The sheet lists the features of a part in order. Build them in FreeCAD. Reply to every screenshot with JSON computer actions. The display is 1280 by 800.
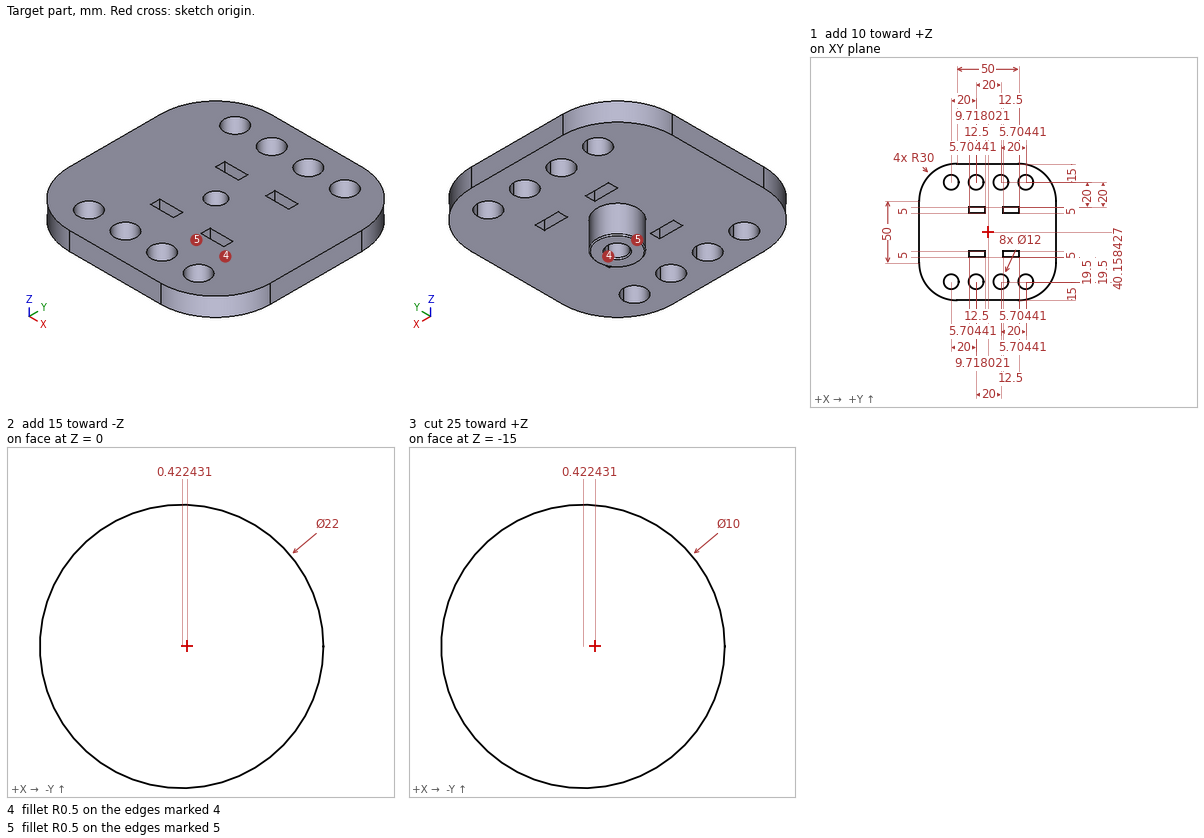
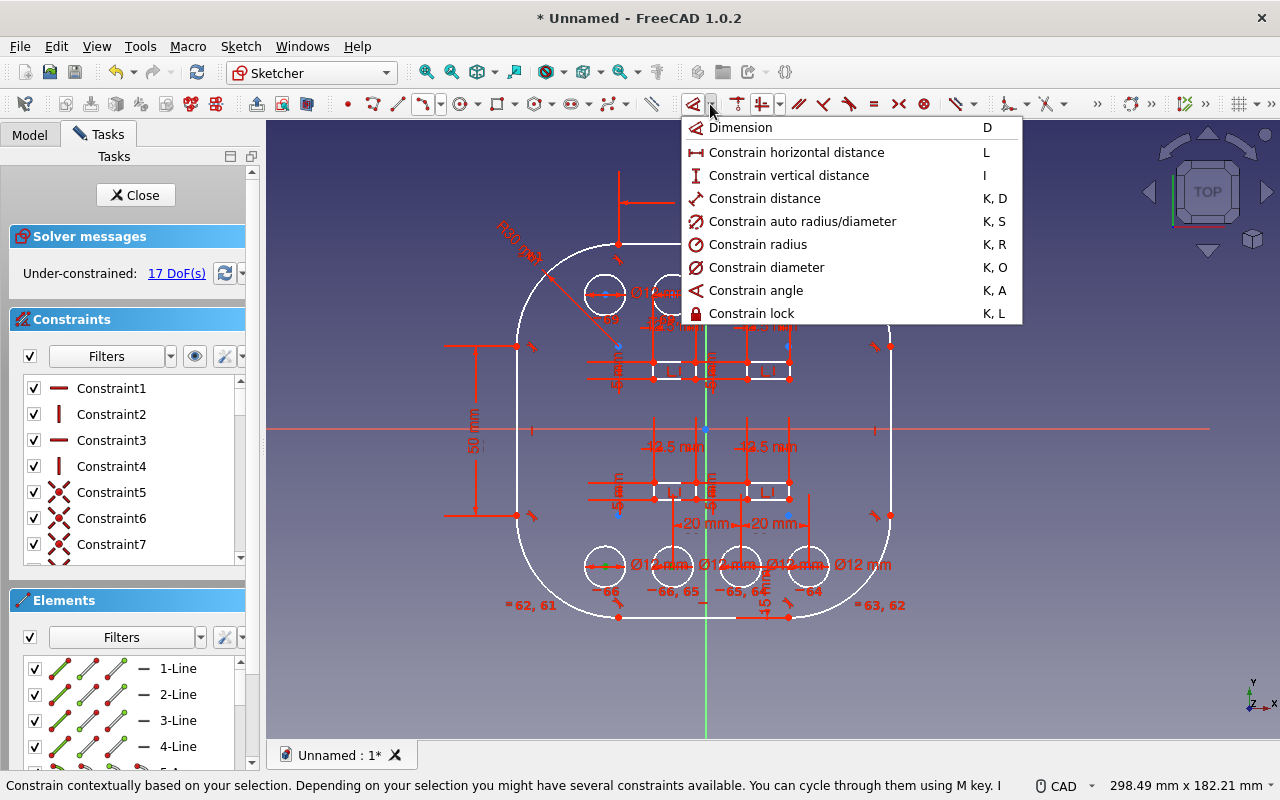
{"action": "left_click", "coordinate": [852, 152]}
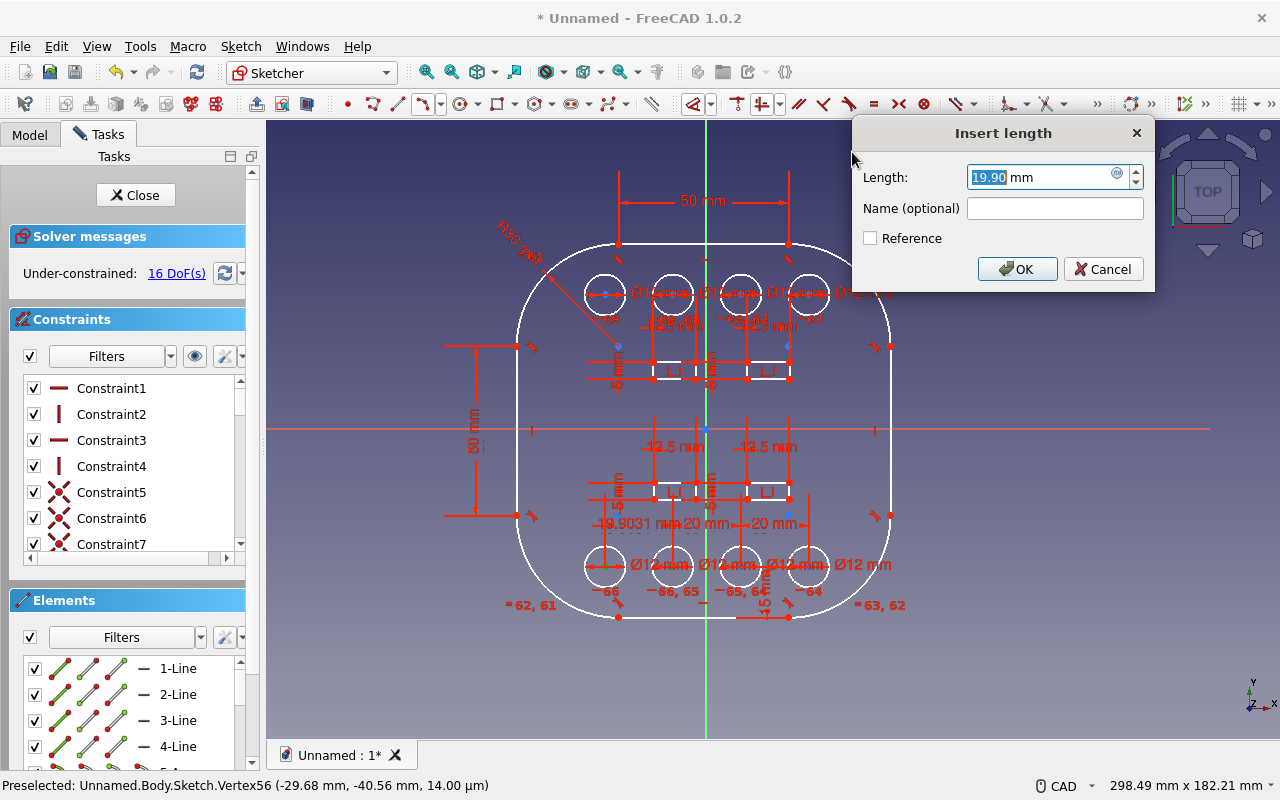
{"action": "type", "text": "20"}
{"action": "key", "text": "Return"}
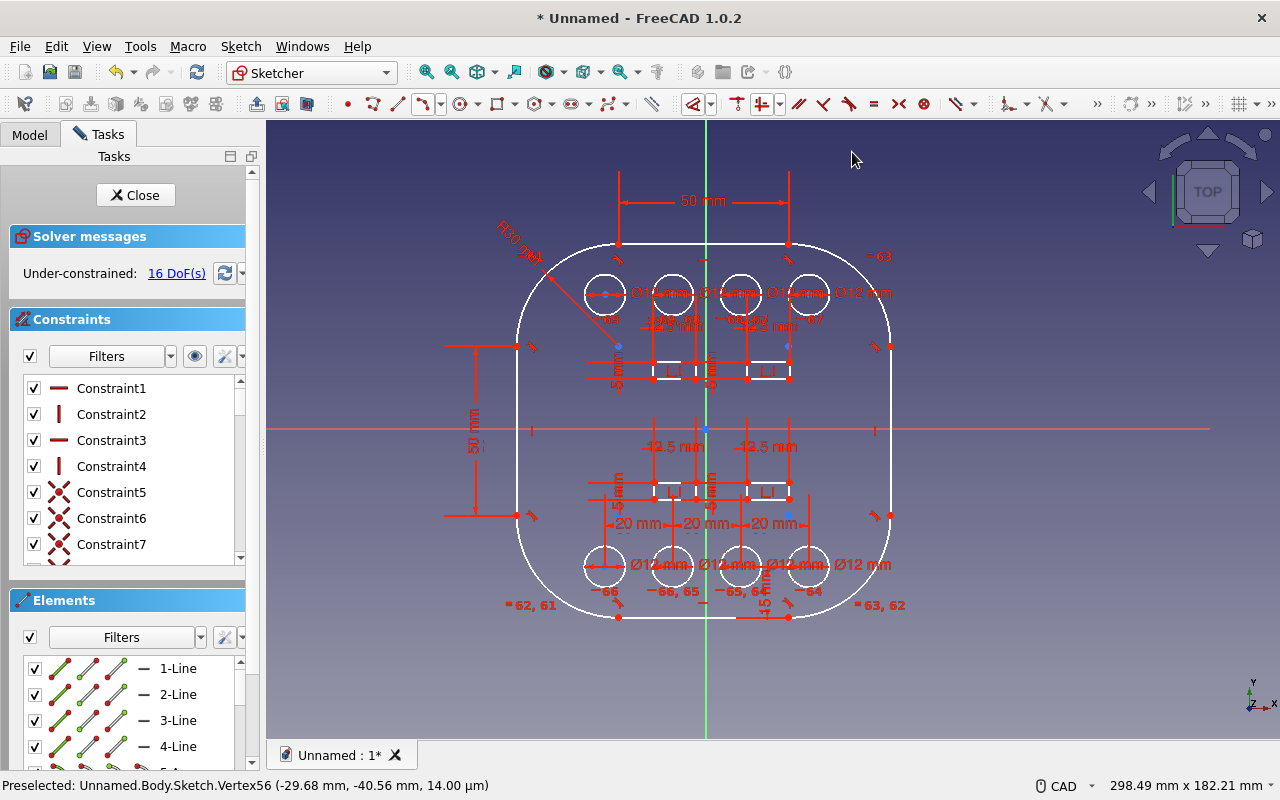
{"action": "left_click", "coordinate": [789, 244]}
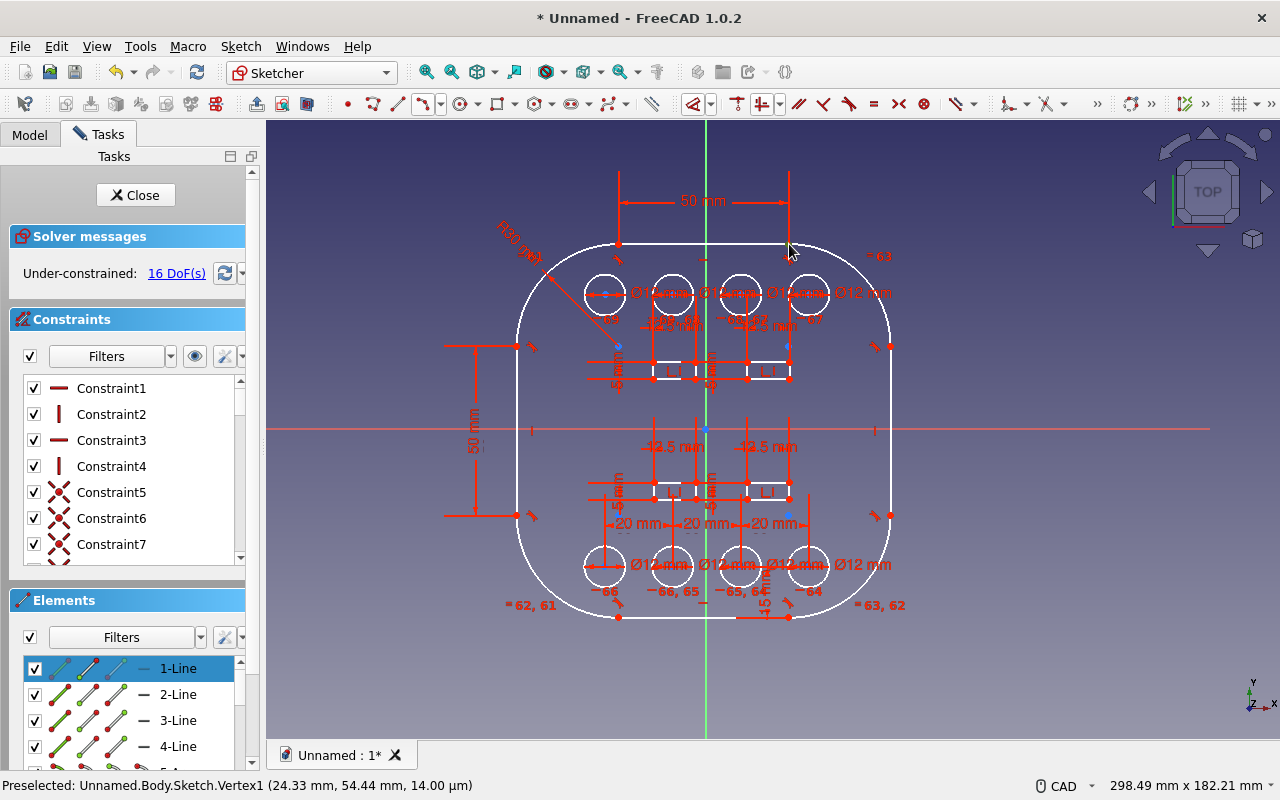
{"action": "left_click", "coordinate": [809, 295]}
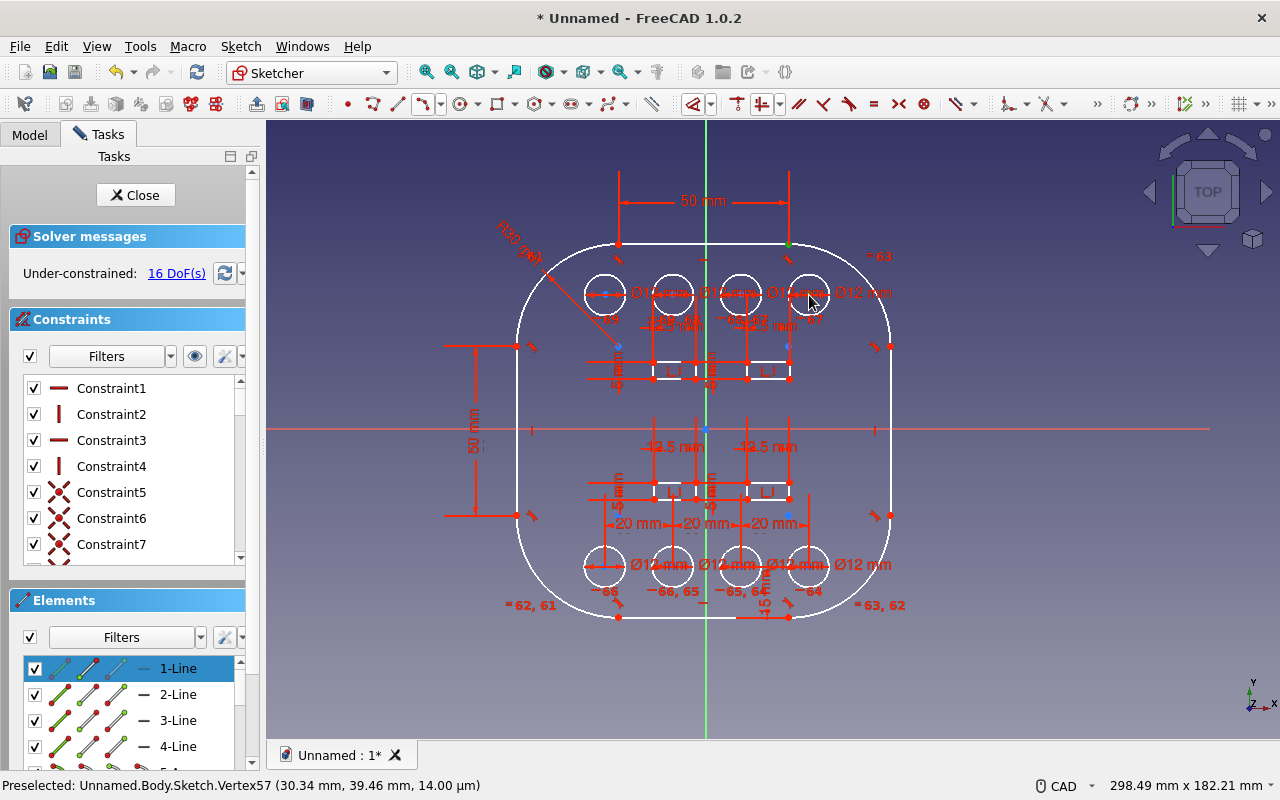
{"action": "left_click", "coordinate": [710, 104]}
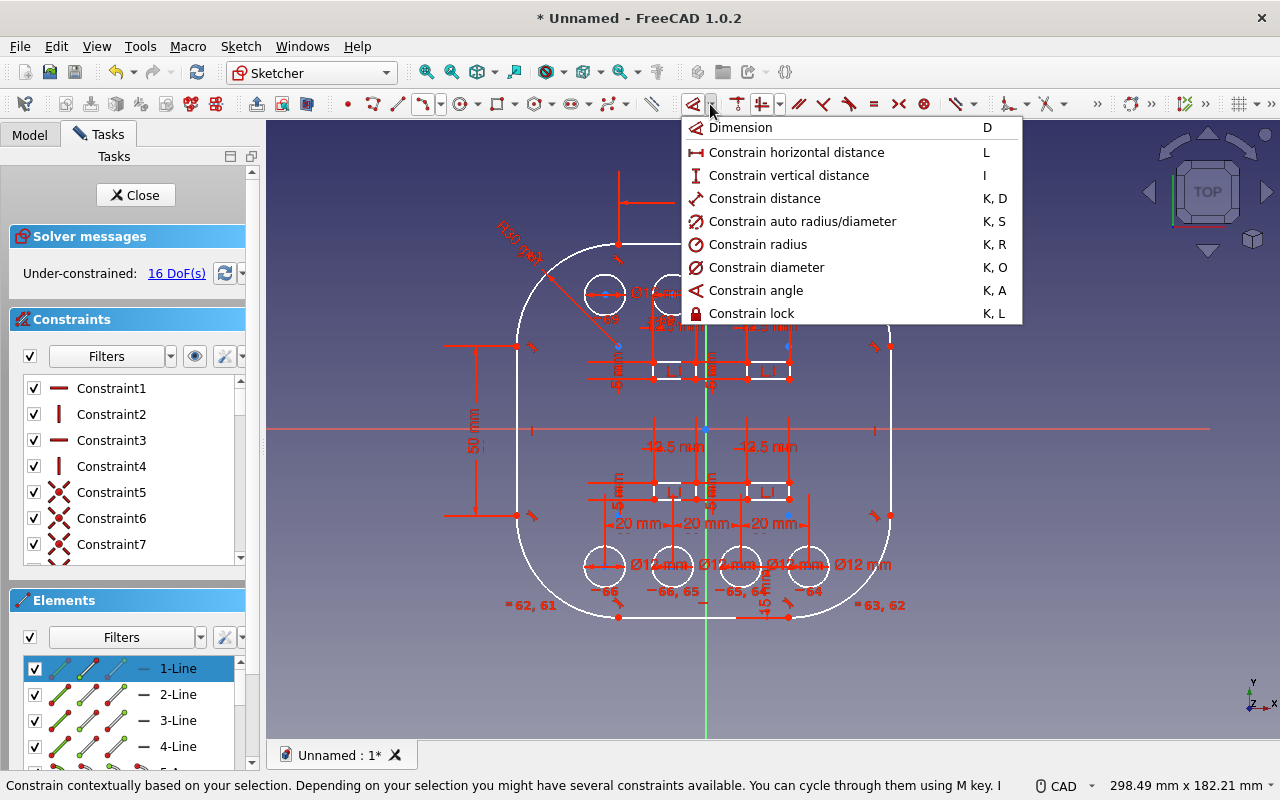
{"action": "left_click", "coordinate": [852, 176]}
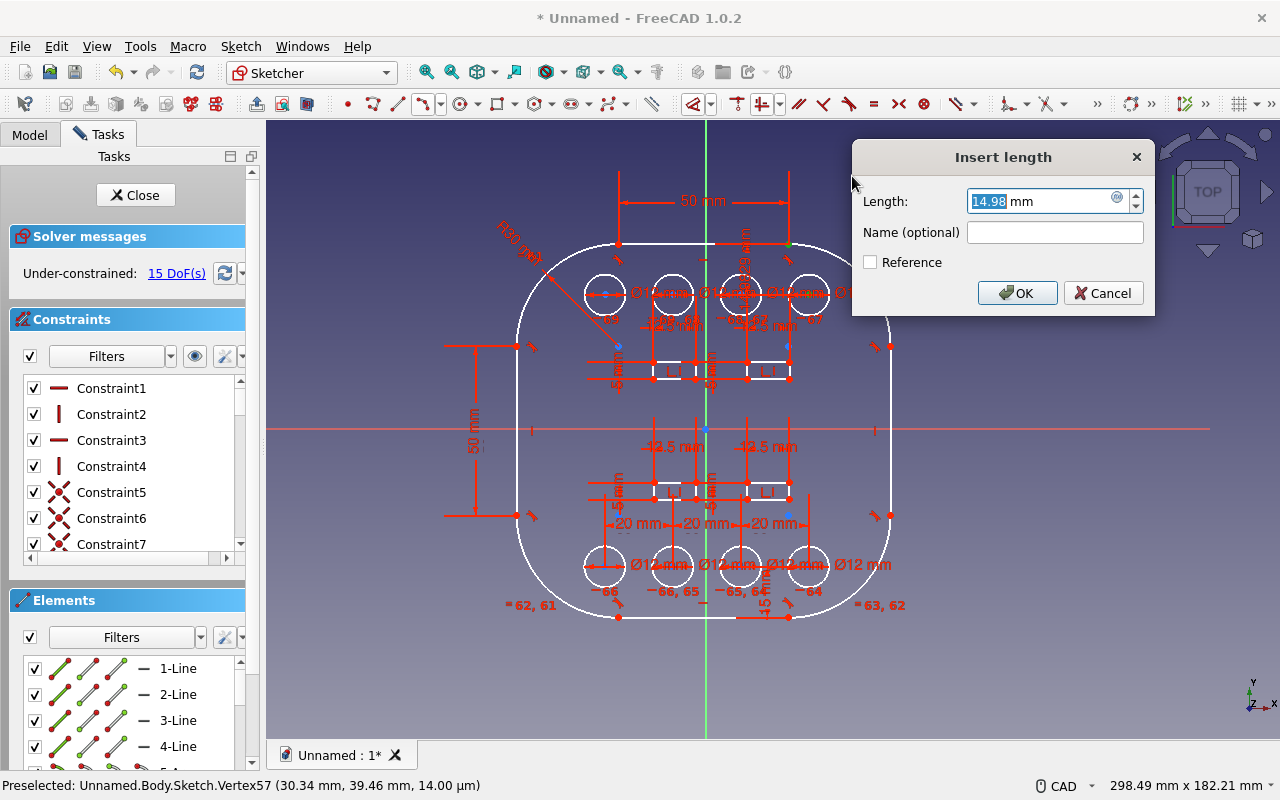
{"action": "type", "text": "15"}
{"action": "key", "text": "Return"}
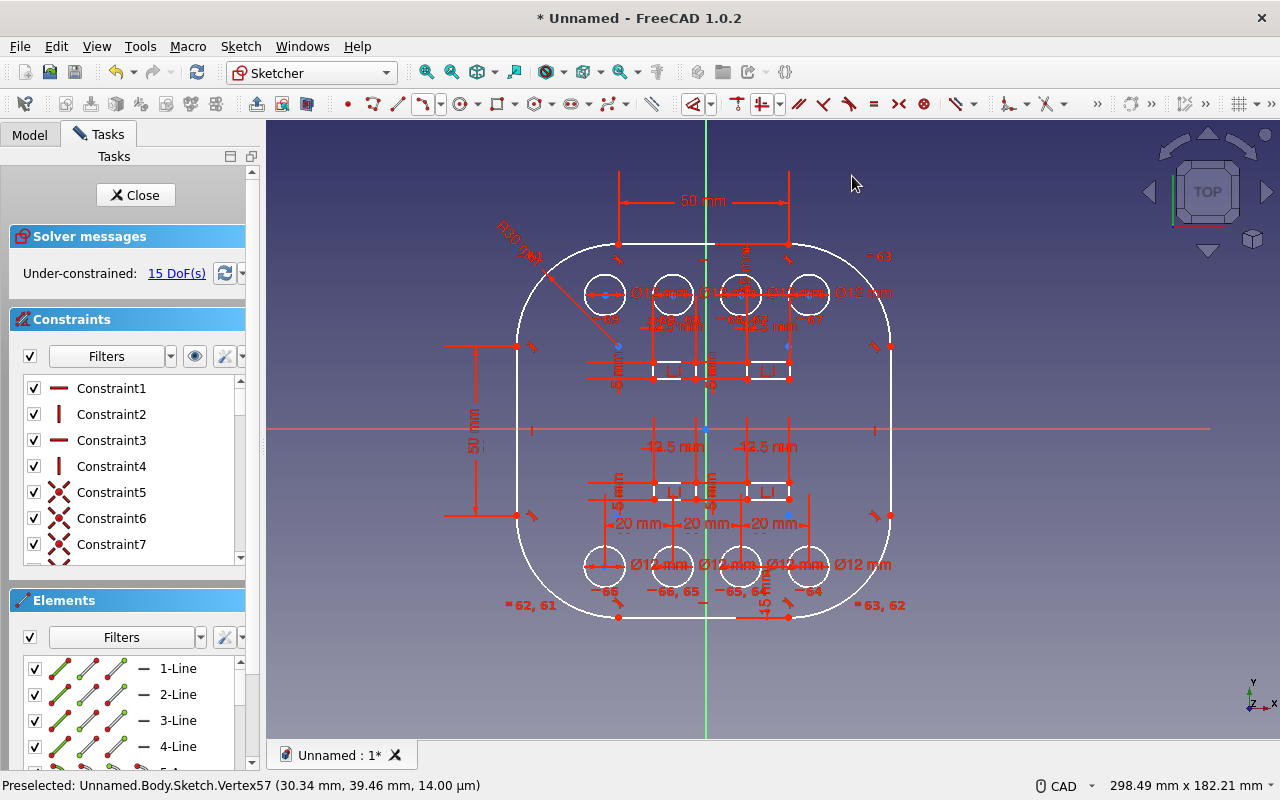
{"action": "left_click", "coordinate": [790, 362]}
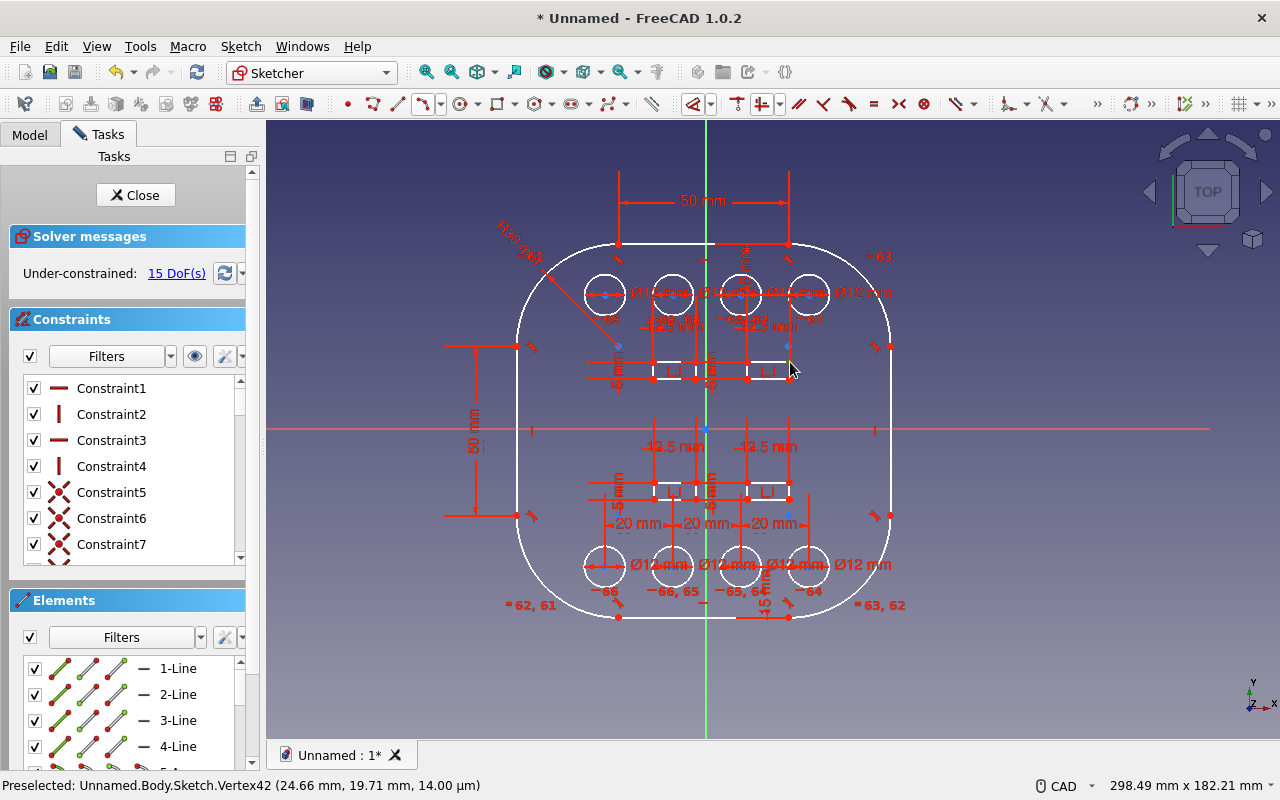
{"action": "left_click", "coordinate": [809, 295]}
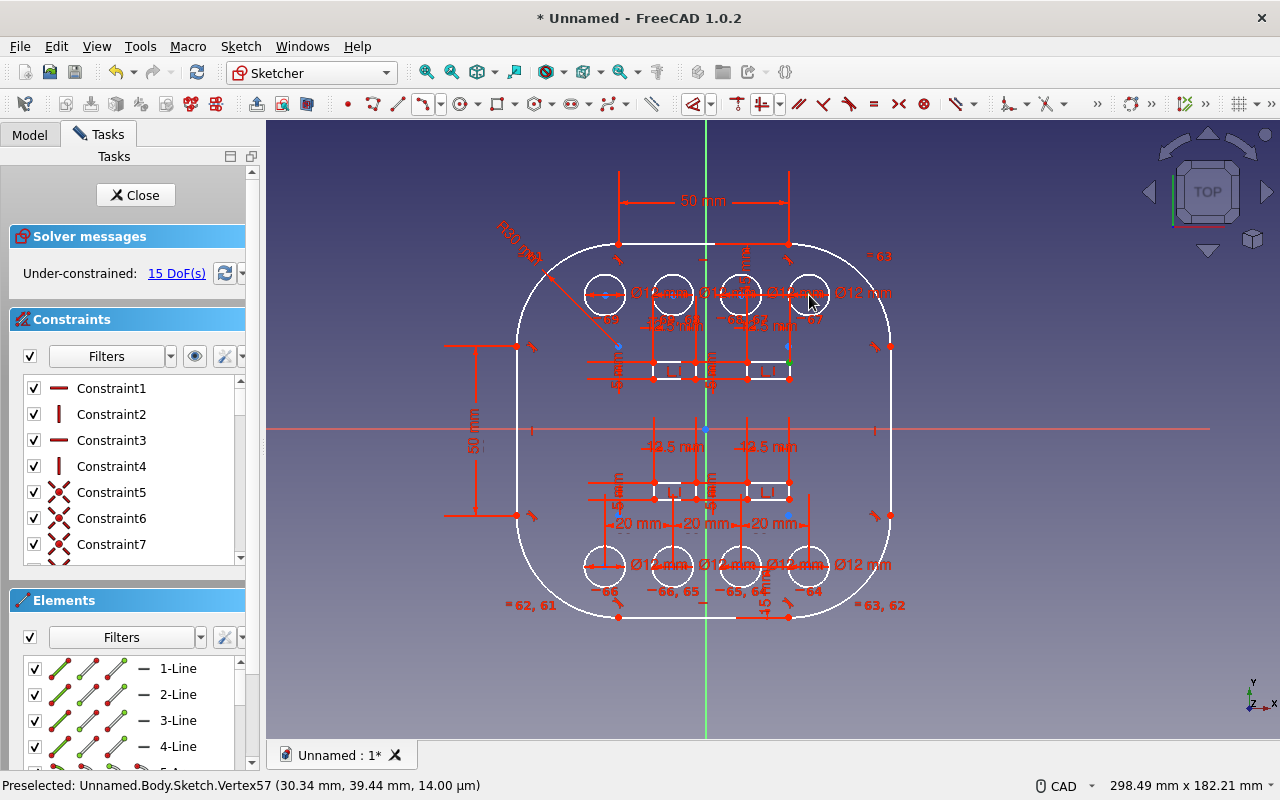
{"action": "key", "text": "i"}